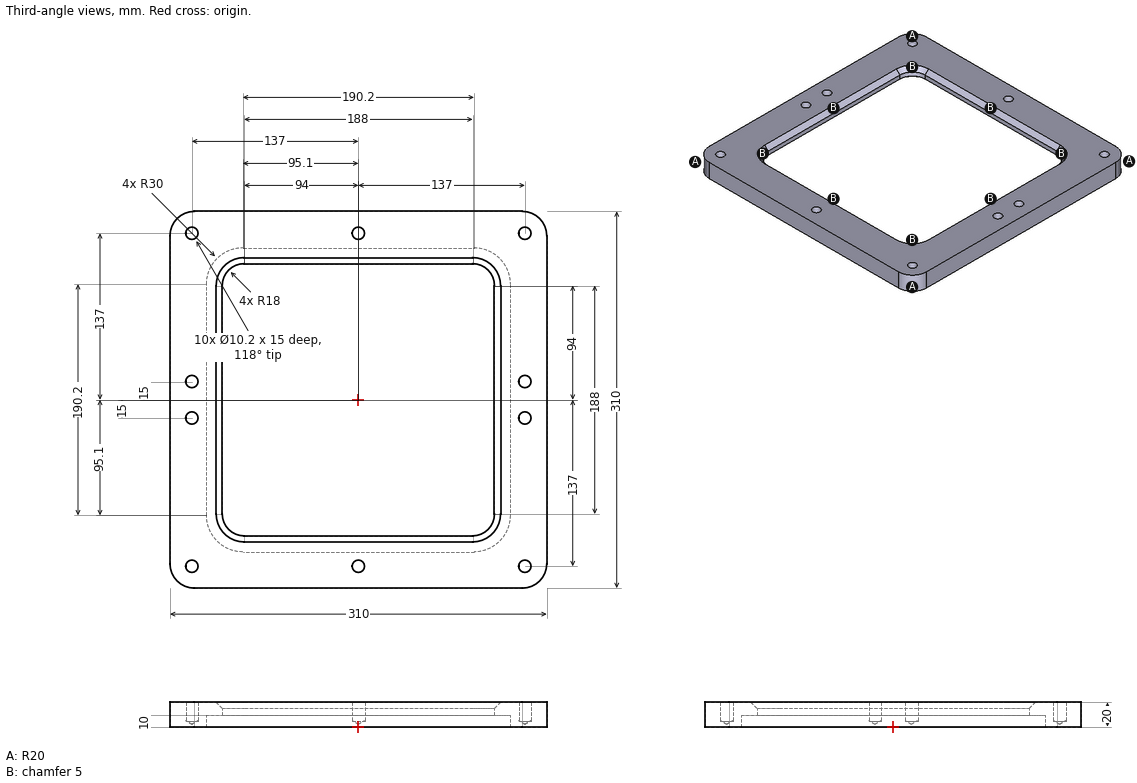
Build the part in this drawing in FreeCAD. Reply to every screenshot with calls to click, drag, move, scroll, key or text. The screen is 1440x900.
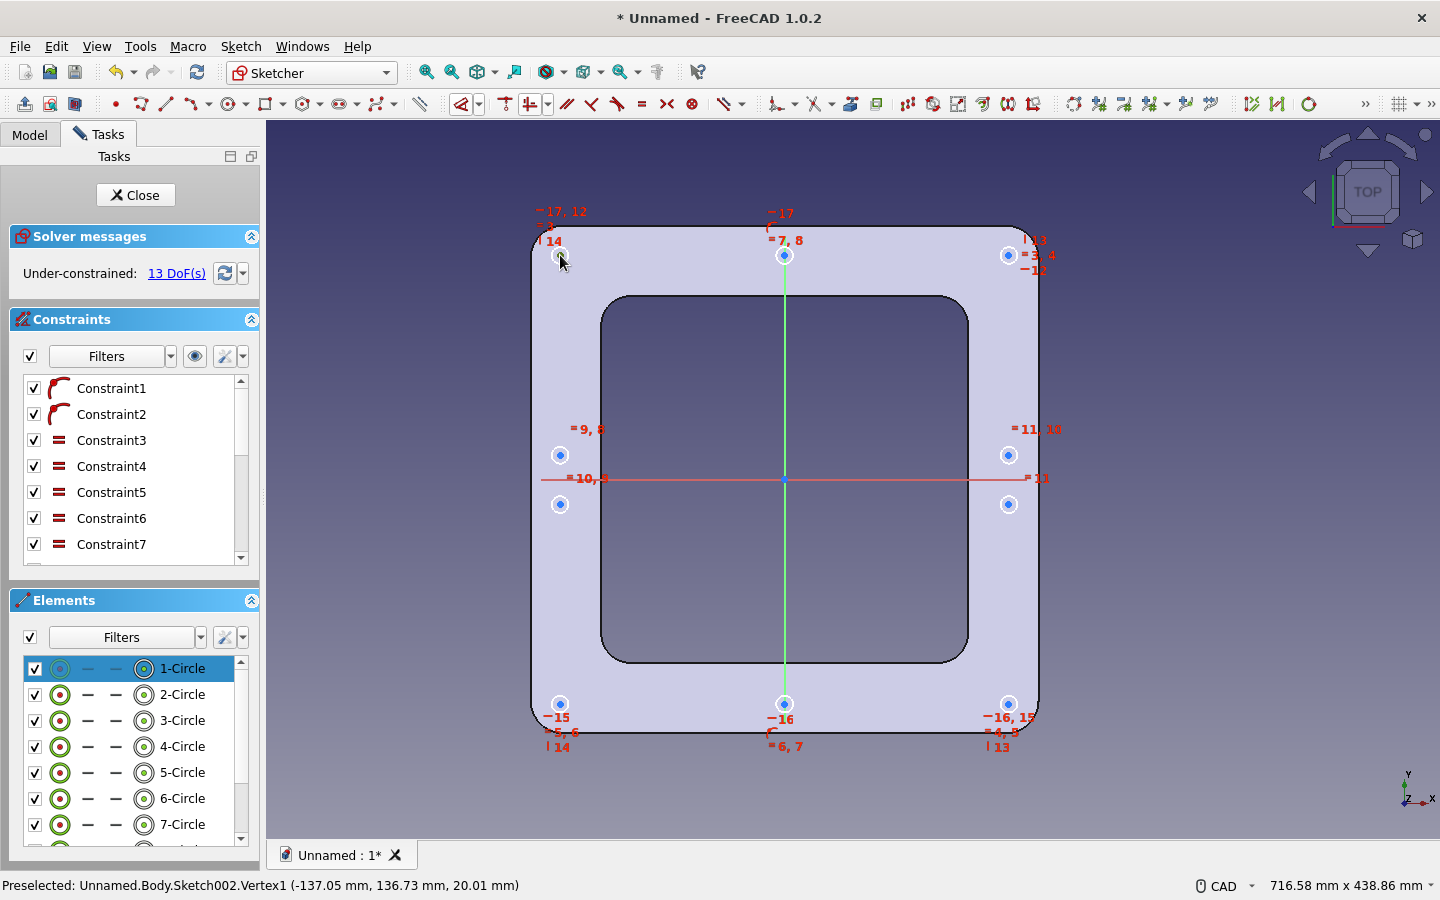
click(560, 455)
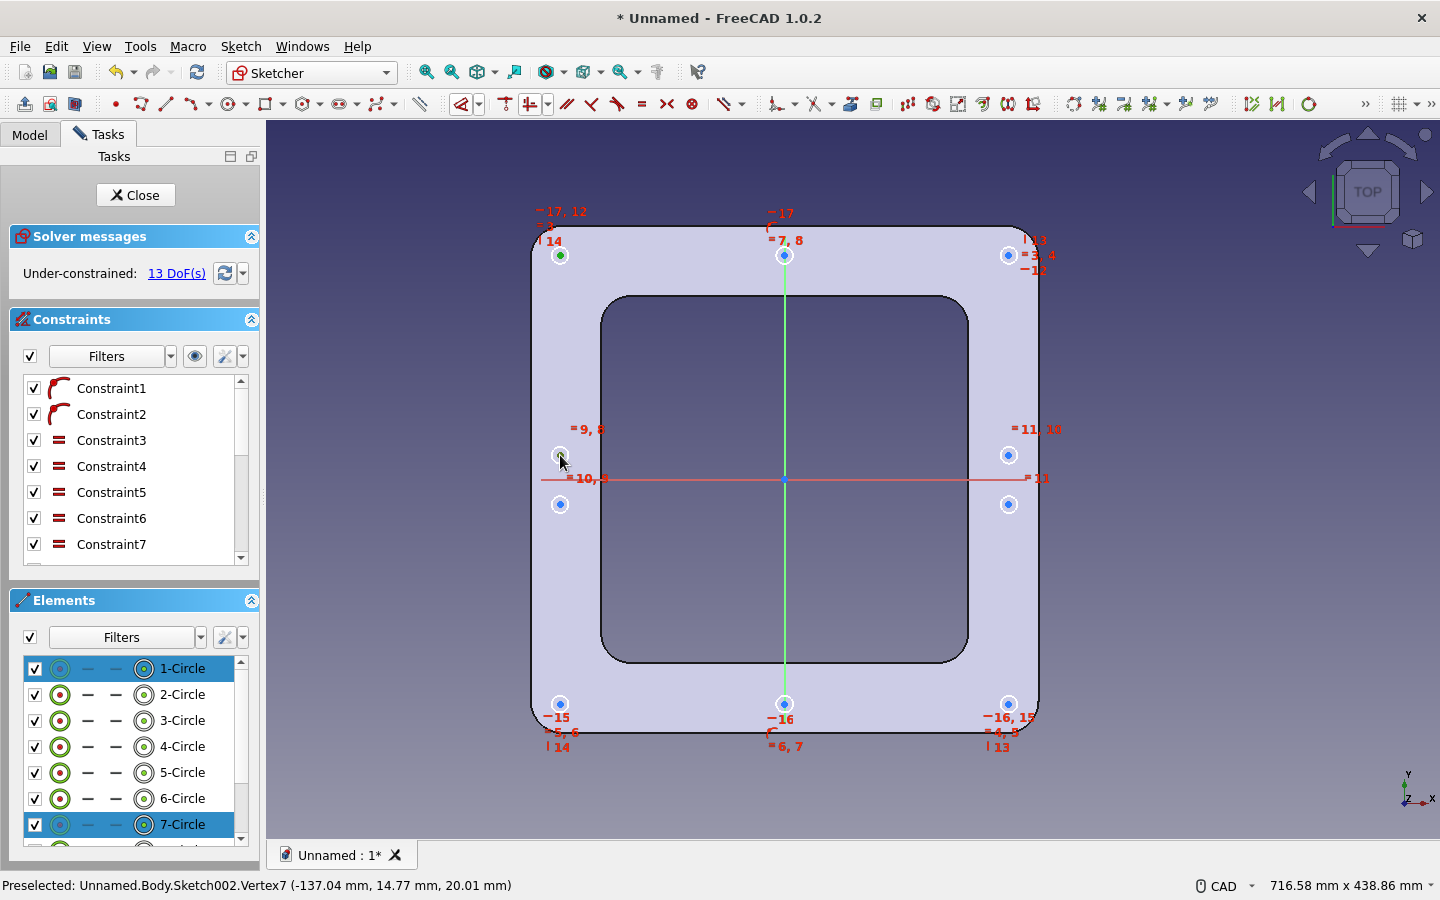
key(v)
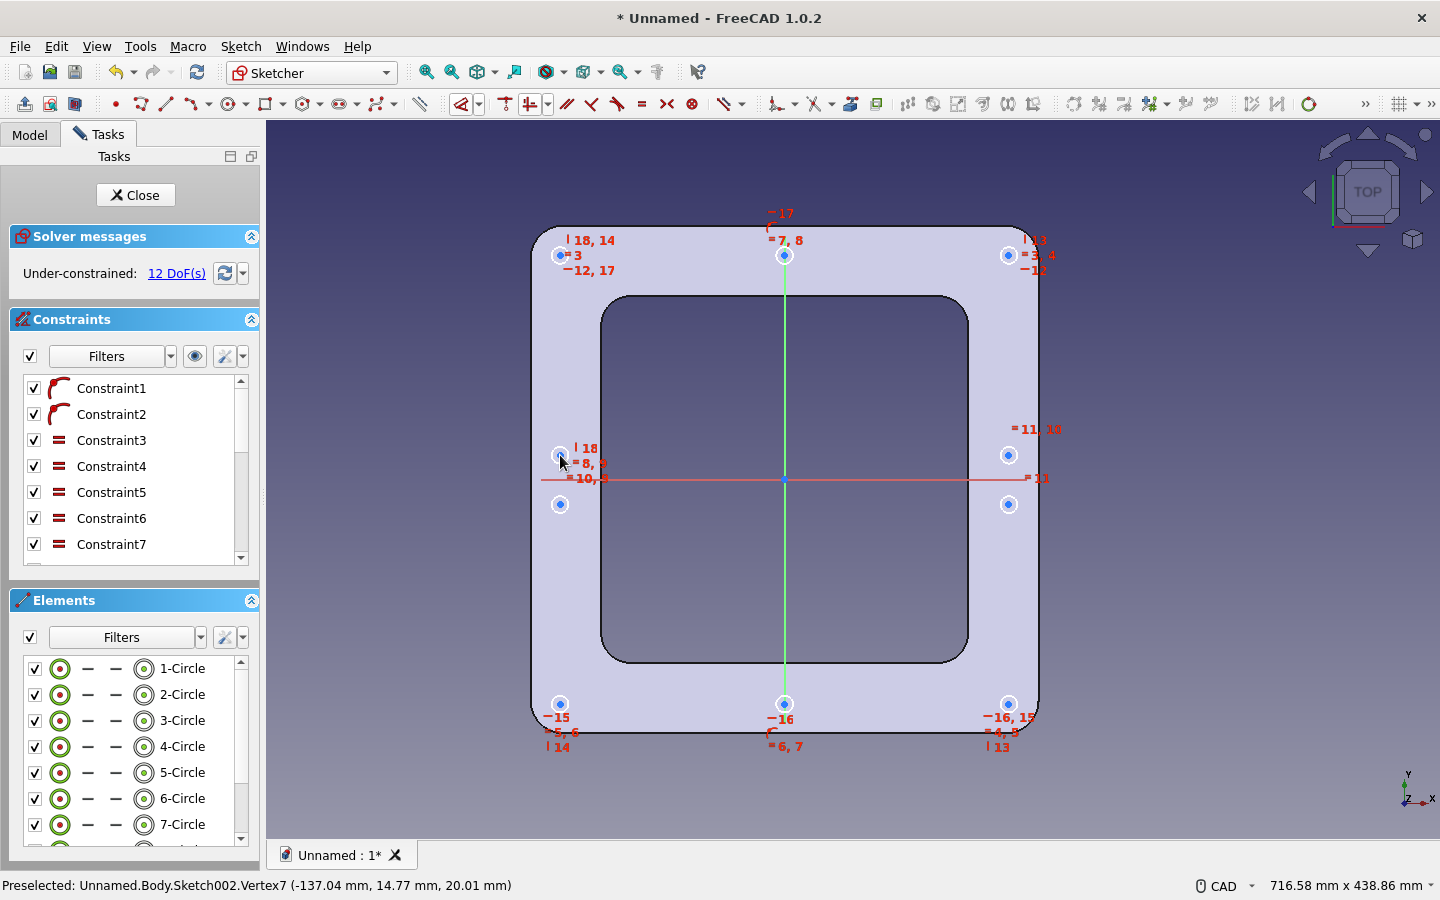
click(560, 455)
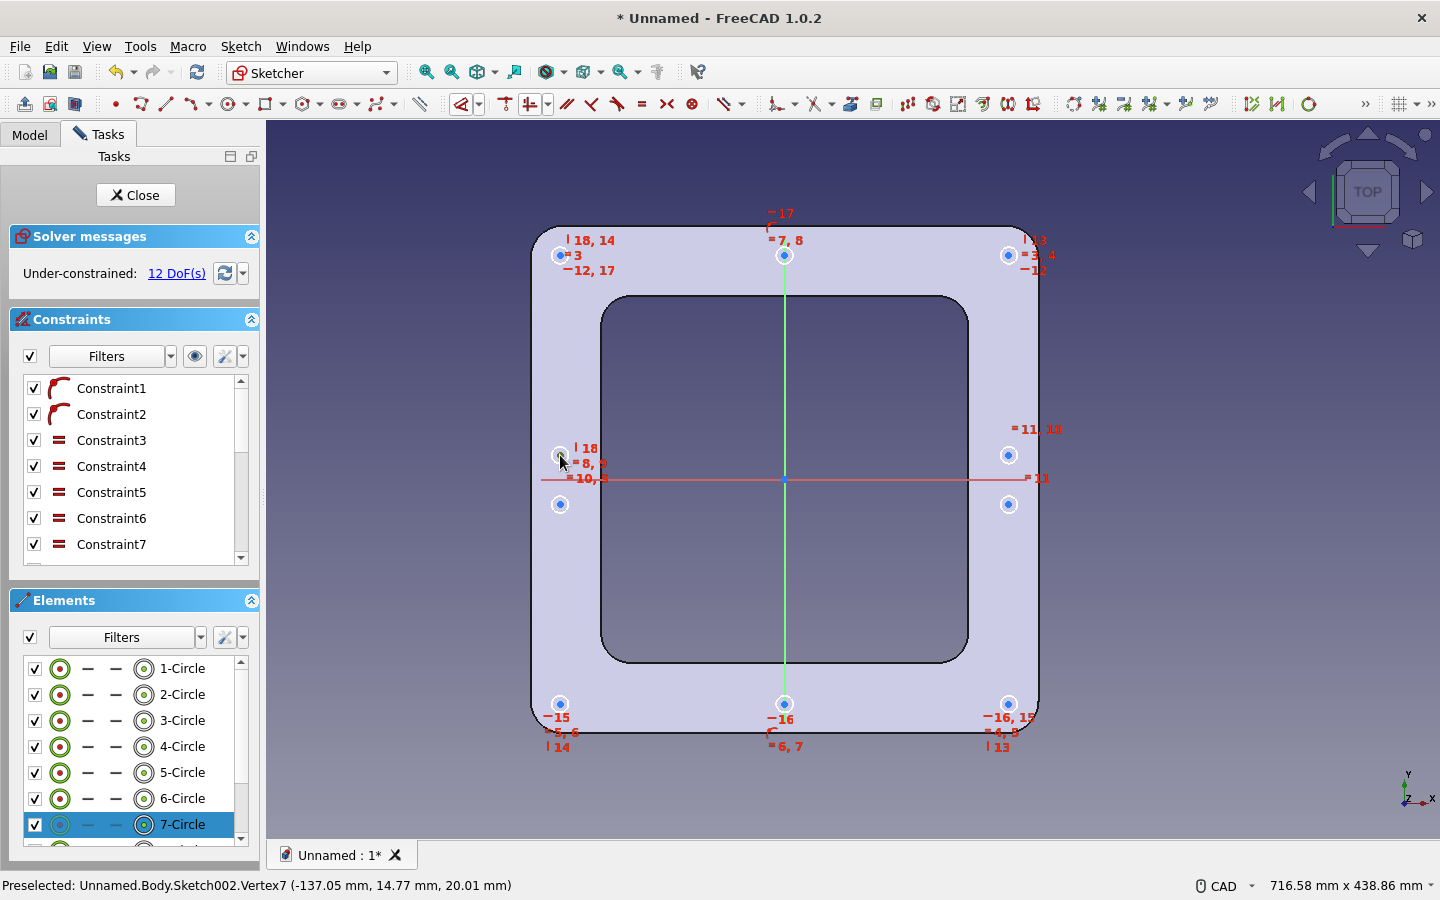
click(560, 505)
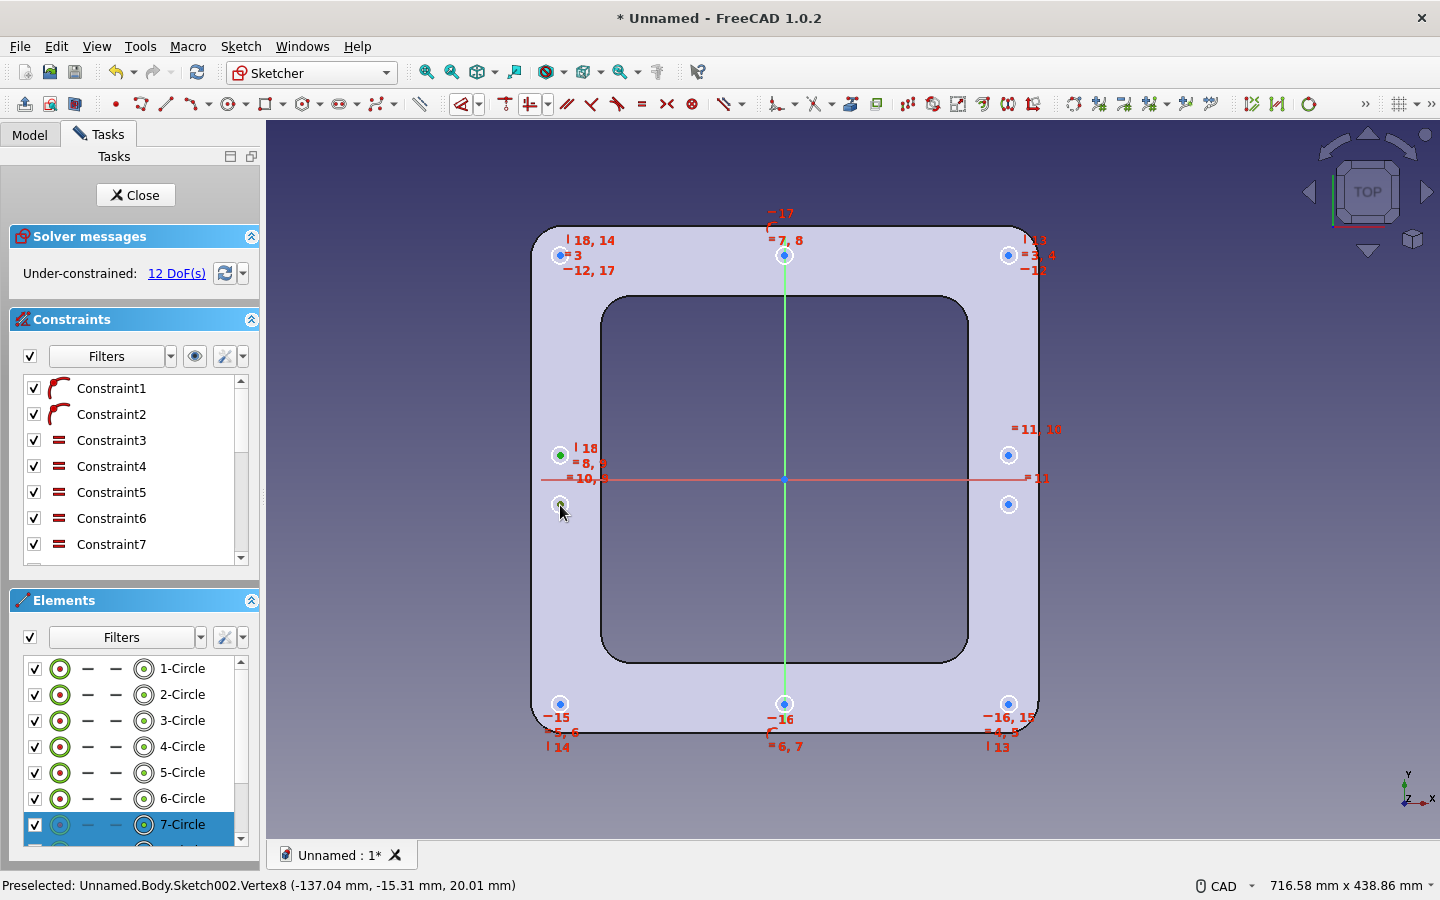
key(v)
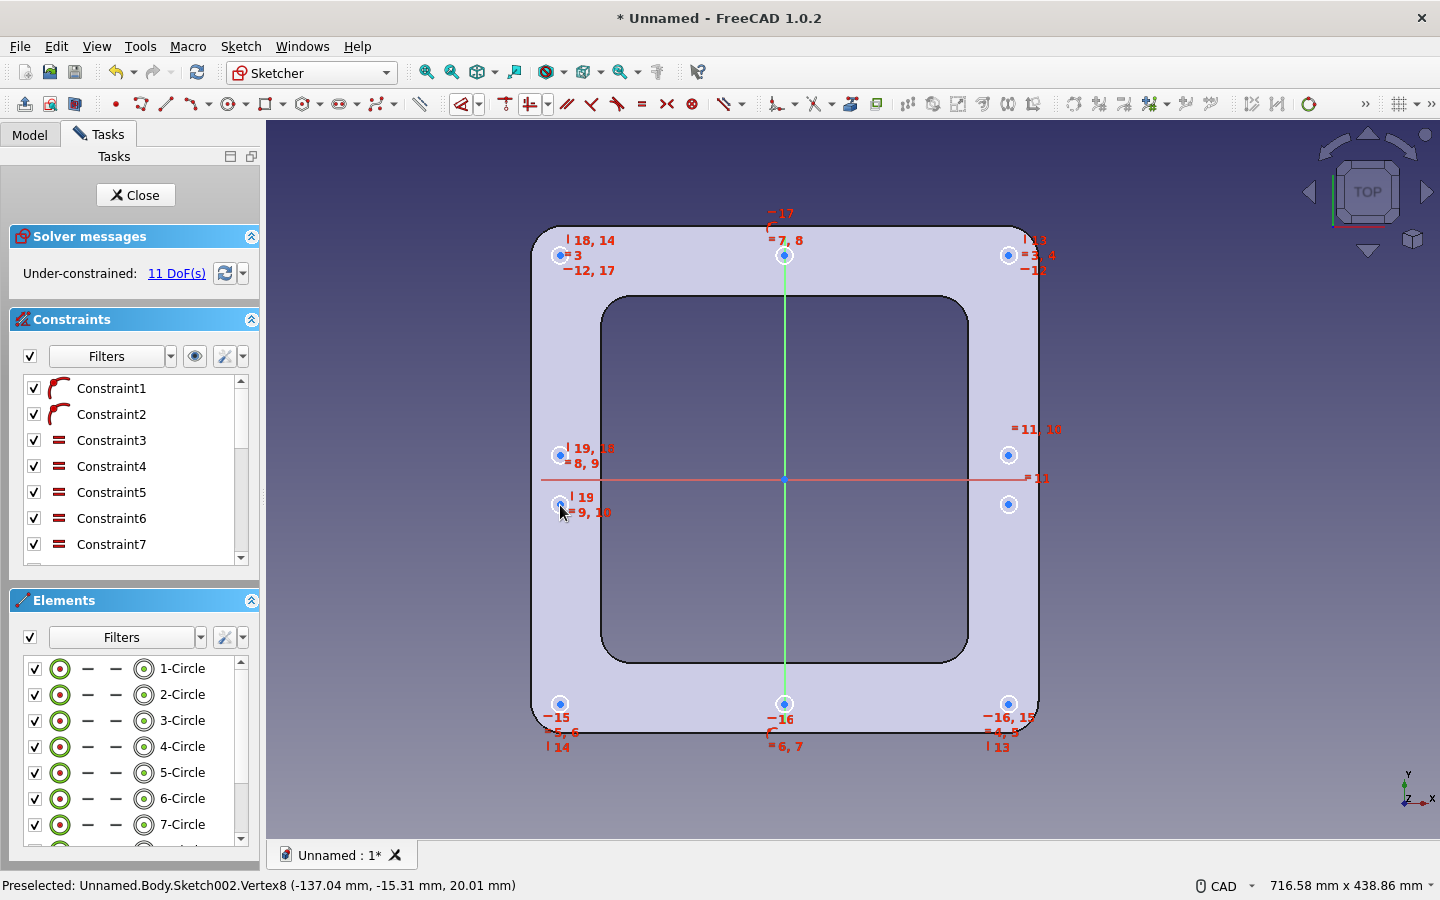
click(1009, 255)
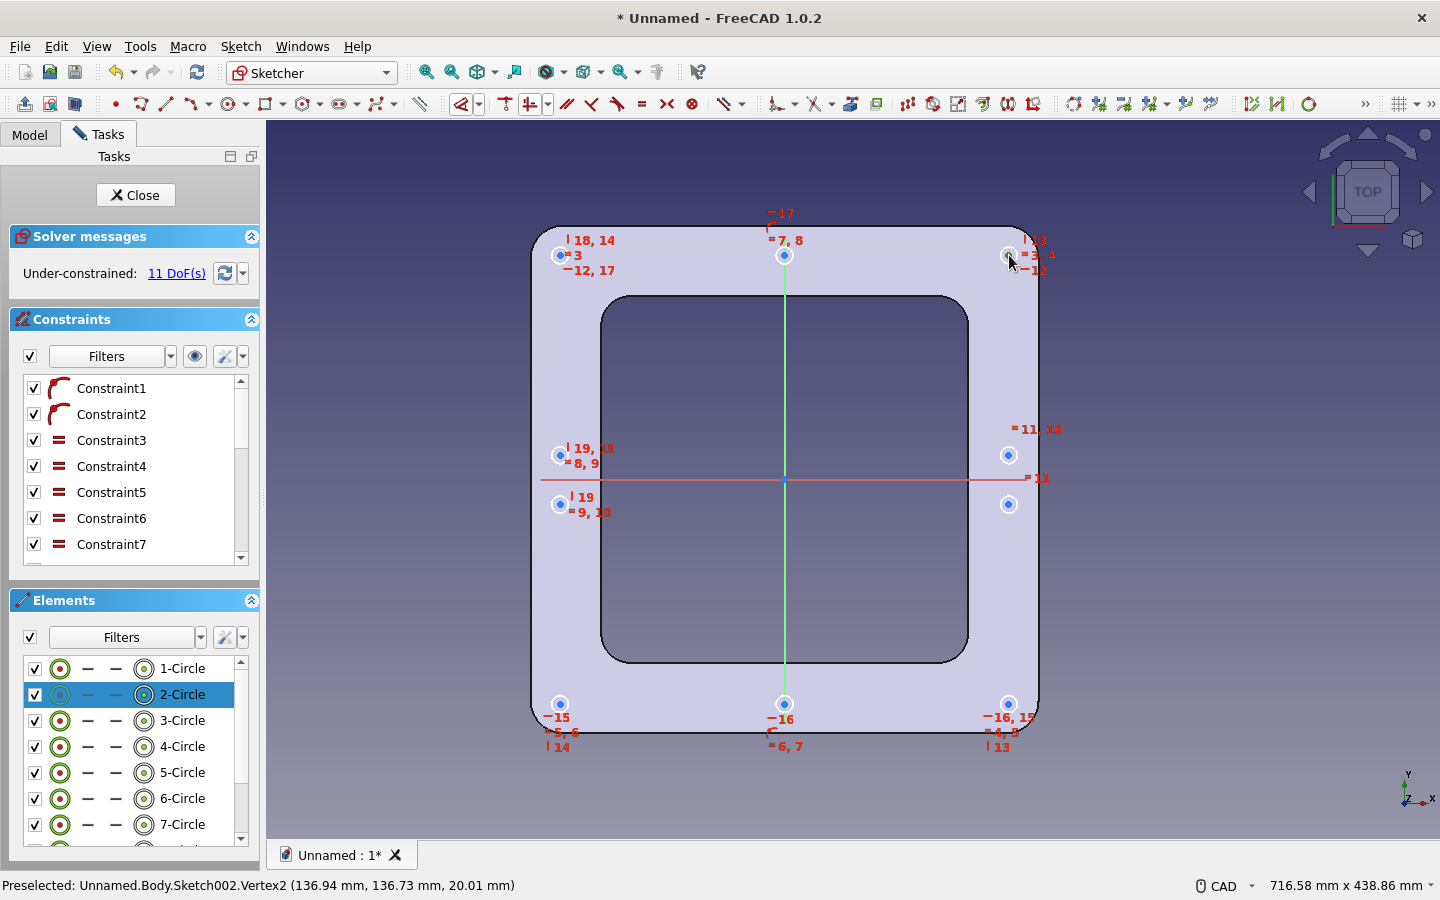
click(1009, 455)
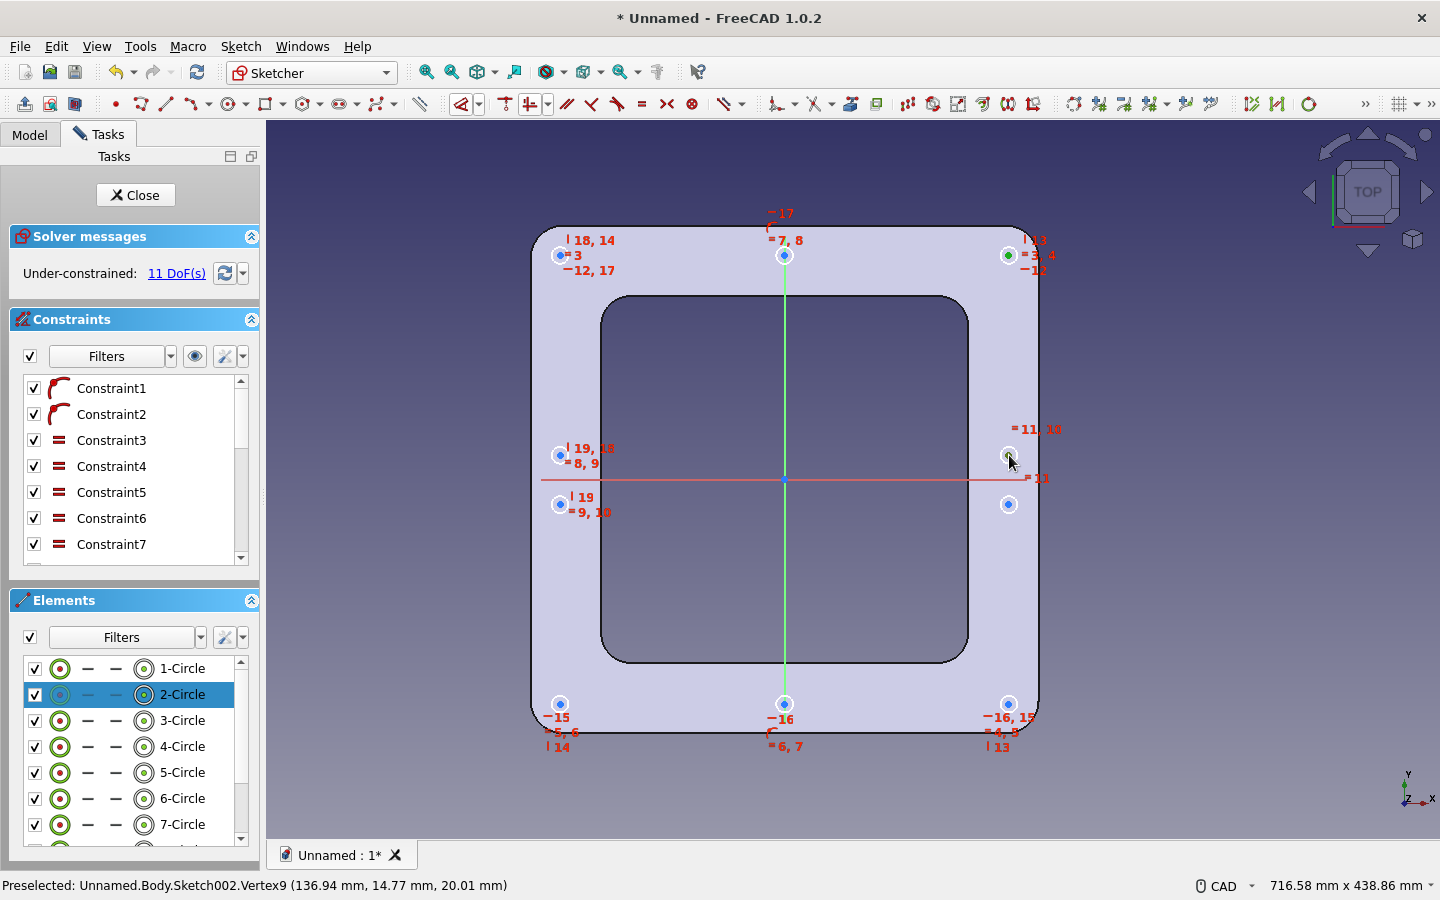
key(v)